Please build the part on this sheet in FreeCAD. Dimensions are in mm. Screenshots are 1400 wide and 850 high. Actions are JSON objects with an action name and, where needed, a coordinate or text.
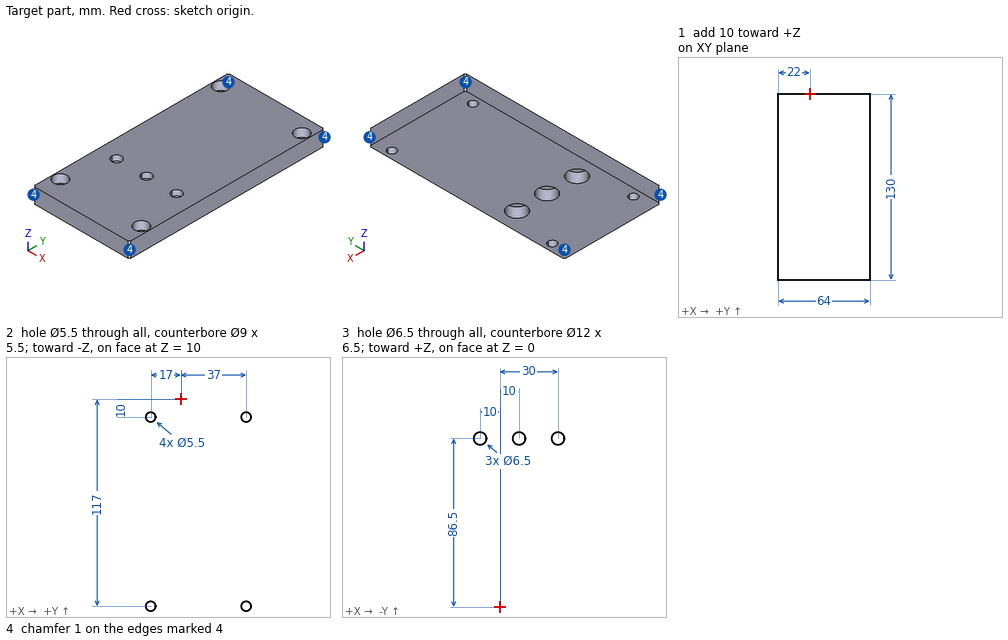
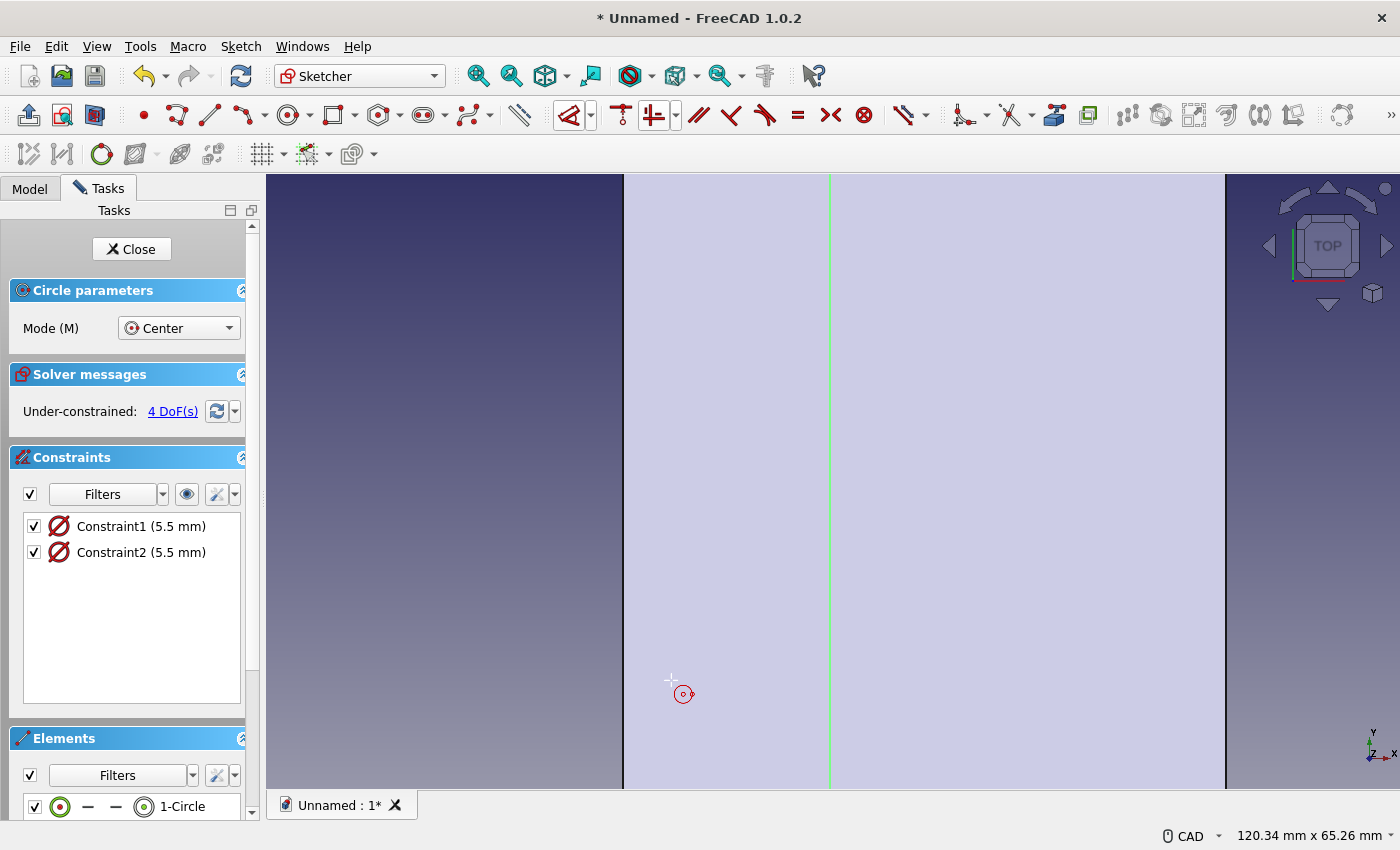
{"action": "left_click", "coordinate": [670, 678]}
{"action": "mouse_move", "coordinate": [688, 660]}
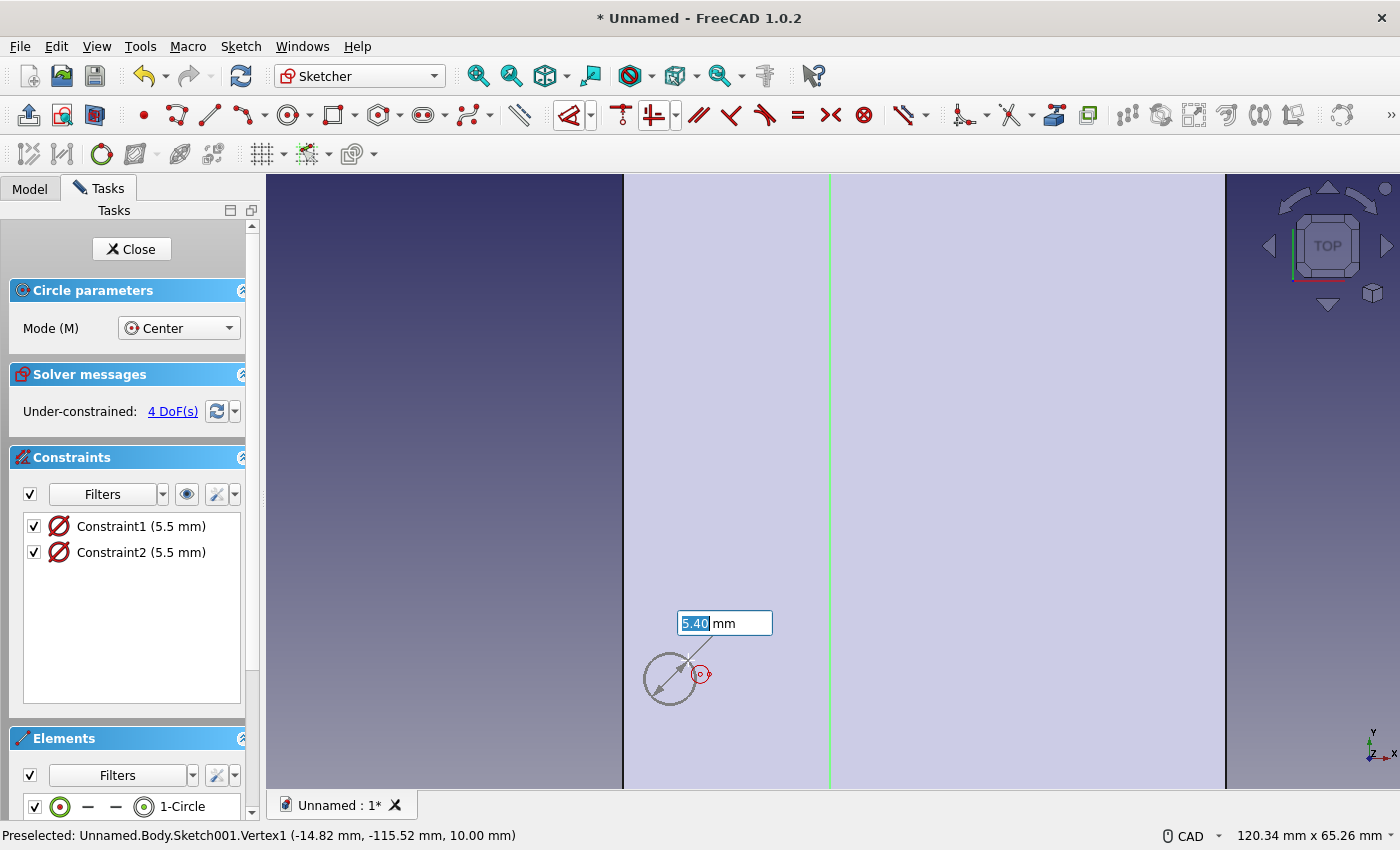
{"action": "type", "text": "5.5"}
{"action": "key", "text": "Return"}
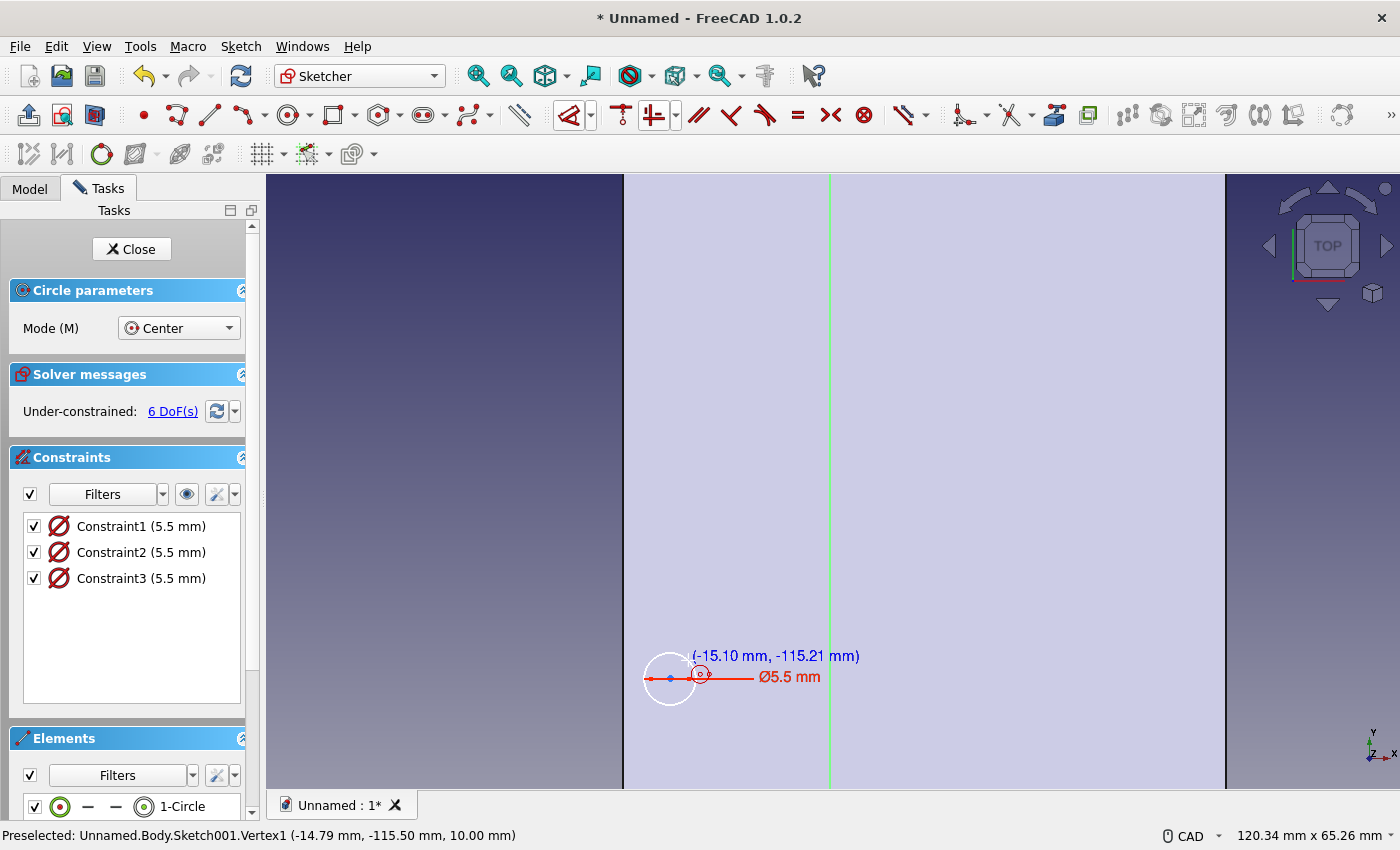
{"action": "left_click", "coordinate": [1179, 678]}
{"action": "mouse_move", "coordinate": [1197, 660]}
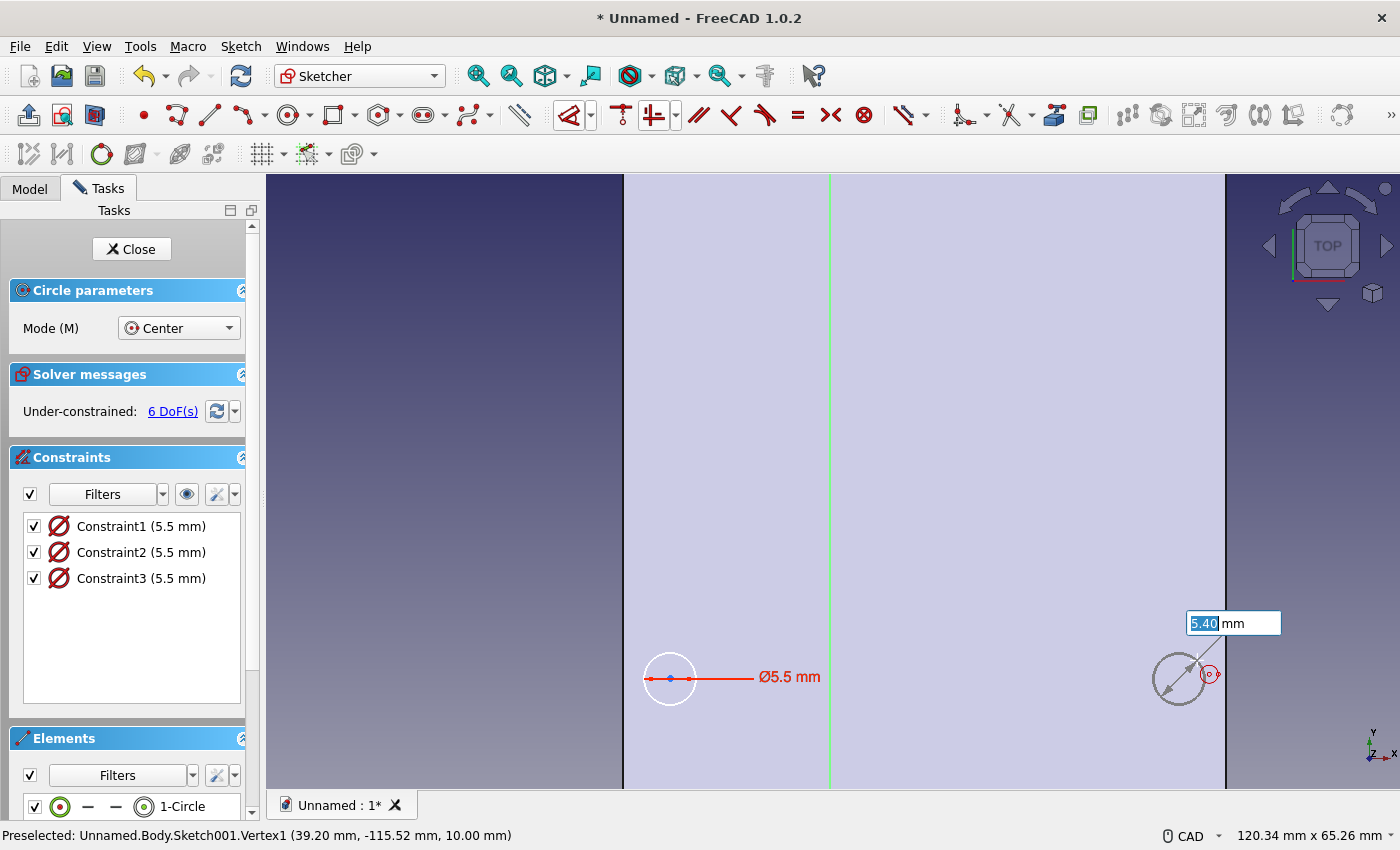
{"action": "type", "text": "5.5"}
{"action": "key", "text": "Return"}
{"action": "key", "text": "Escape"}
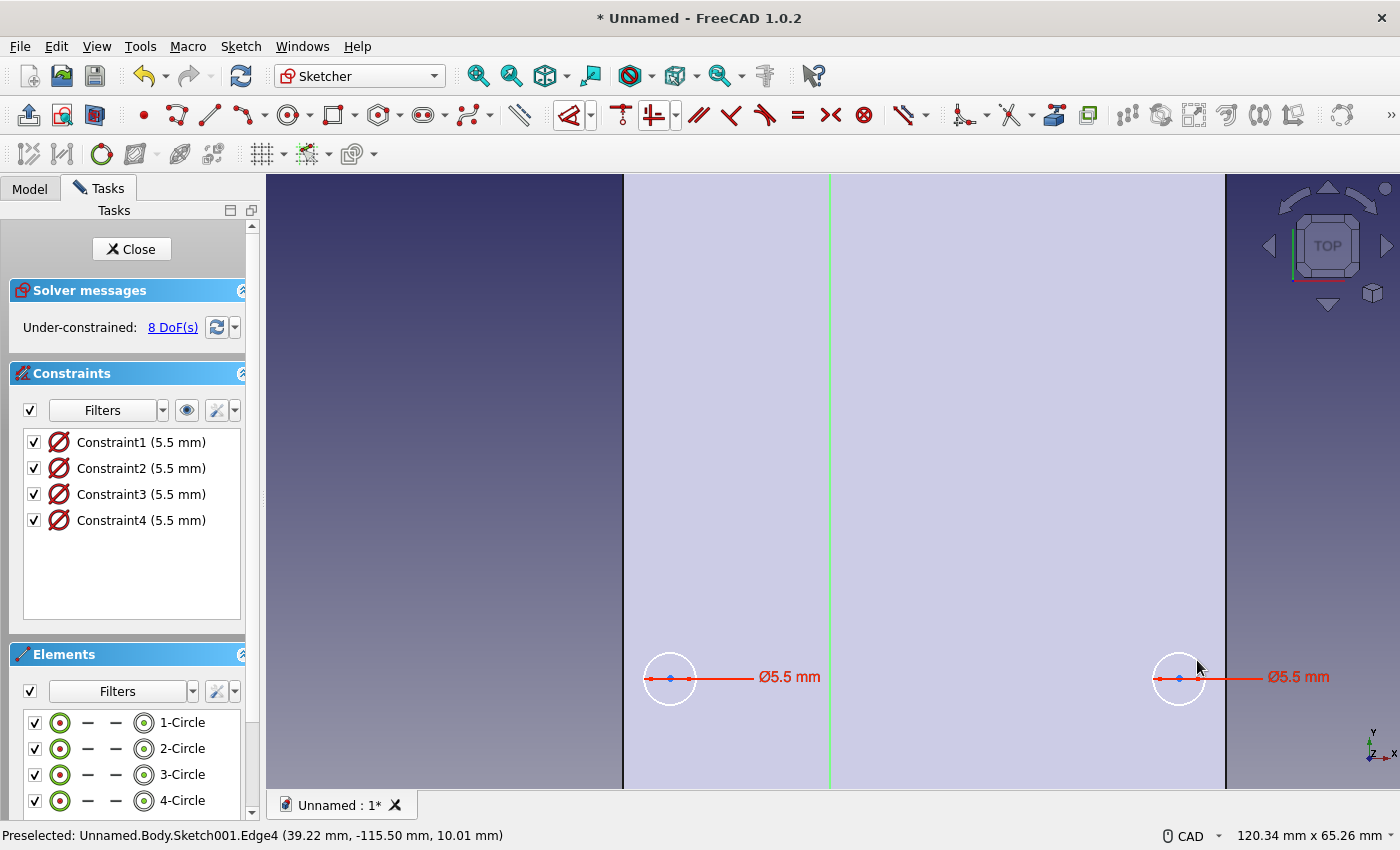
{"action": "scroll", "coordinate": [671, 680], "scroll_direction": "down", "scroll_amount": 5}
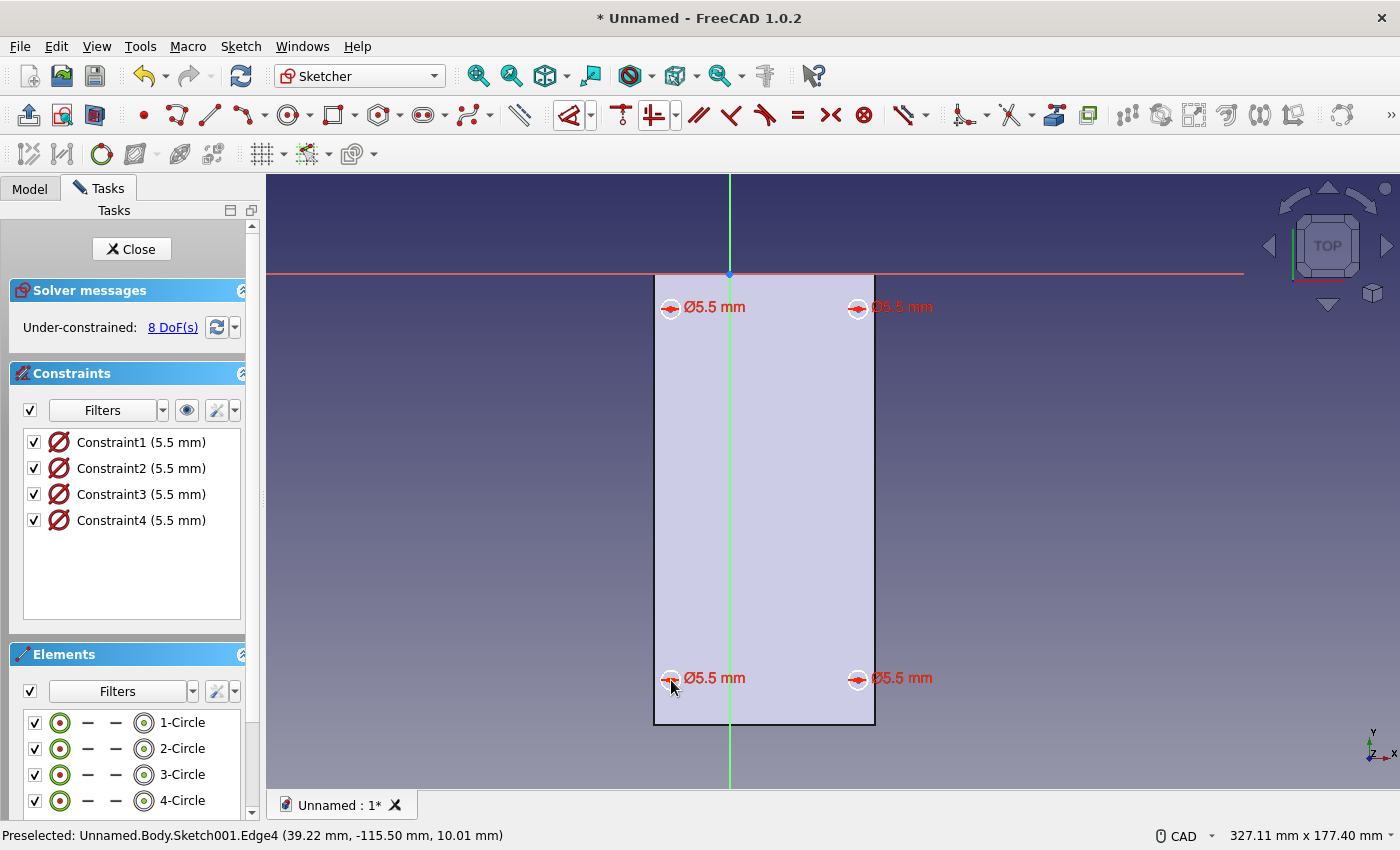
{"action": "left_click", "coordinate": [671, 309]}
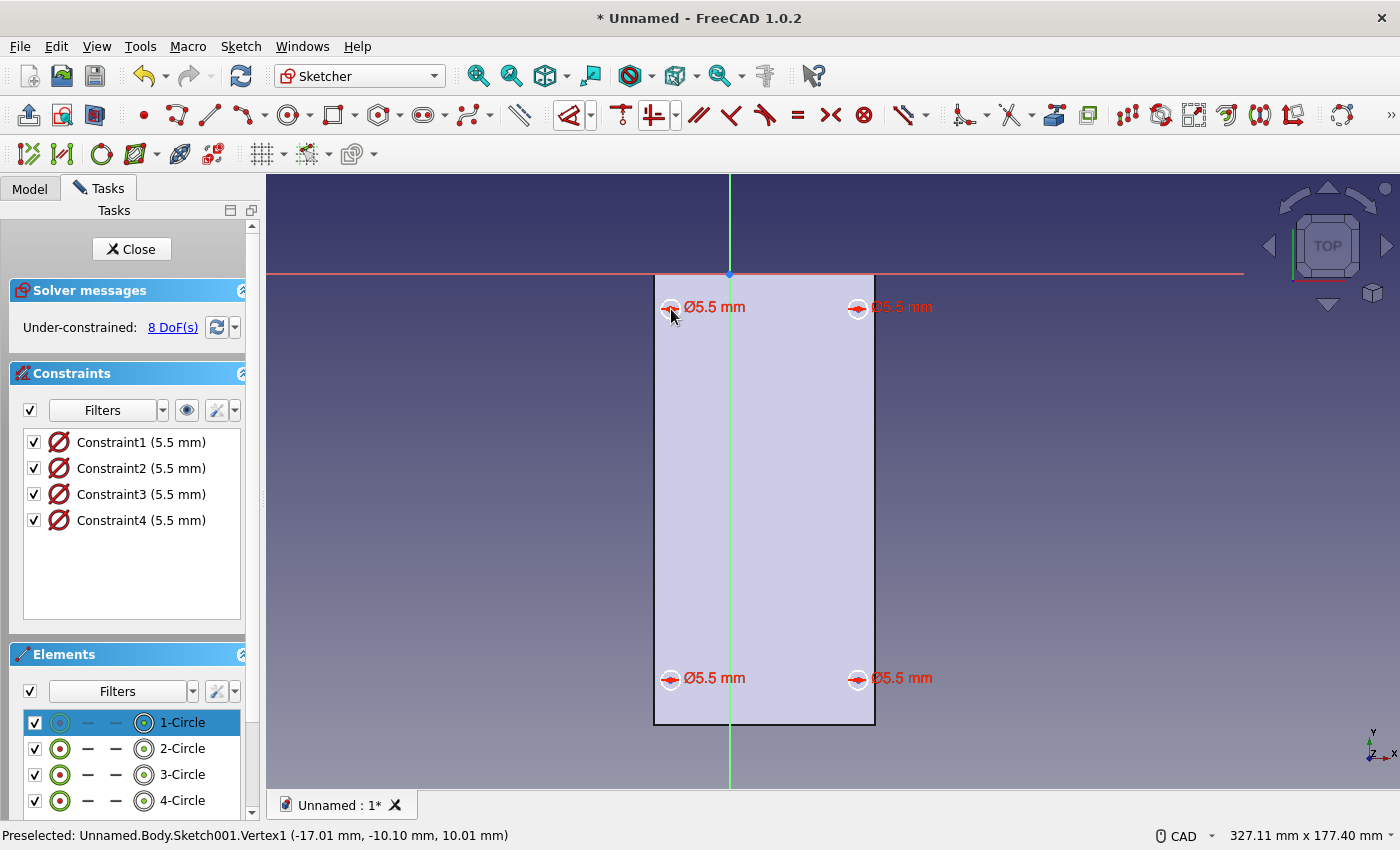
{"action": "left_click", "coordinate": [858, 309]}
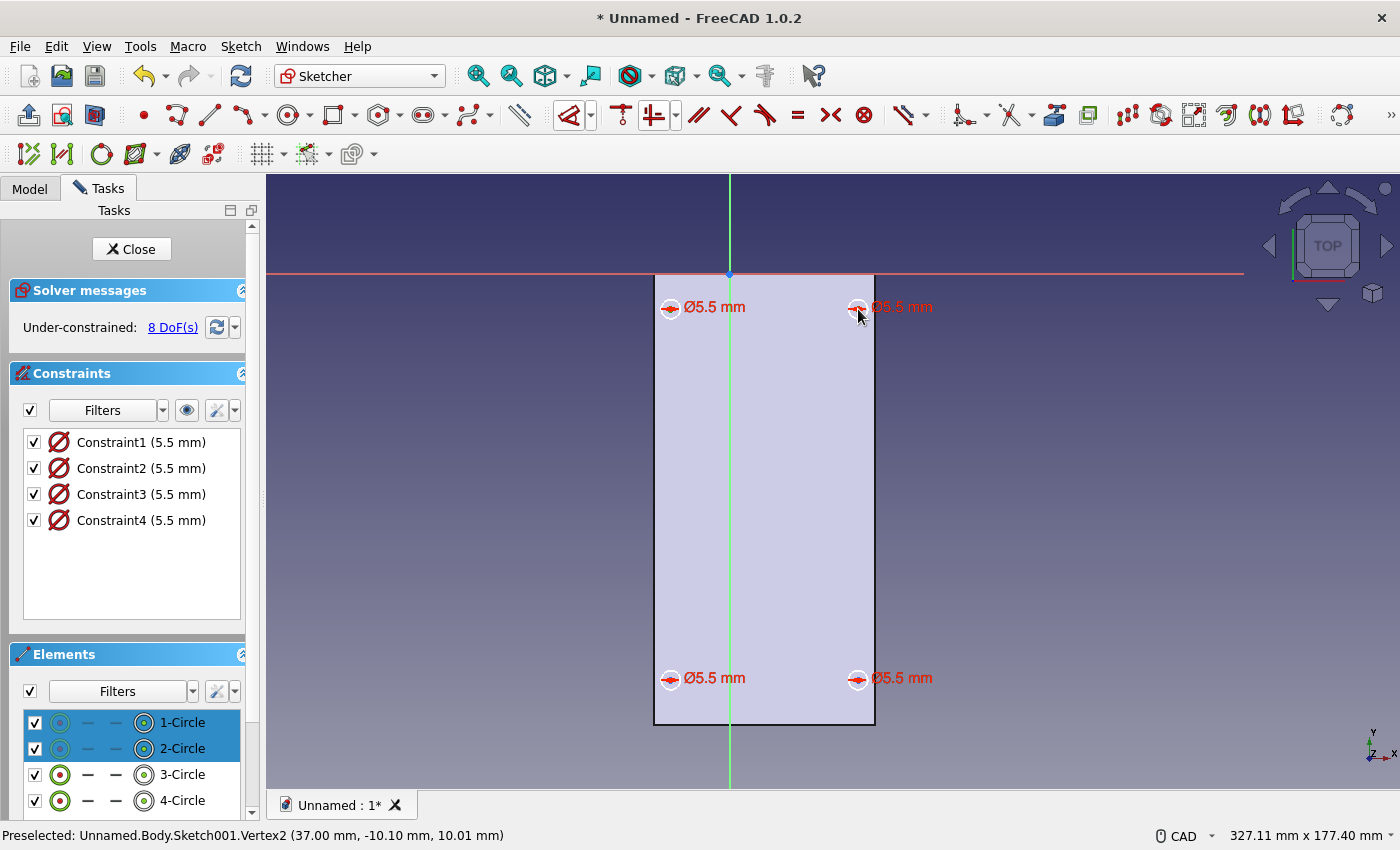
{"action": "key", "text": "h"}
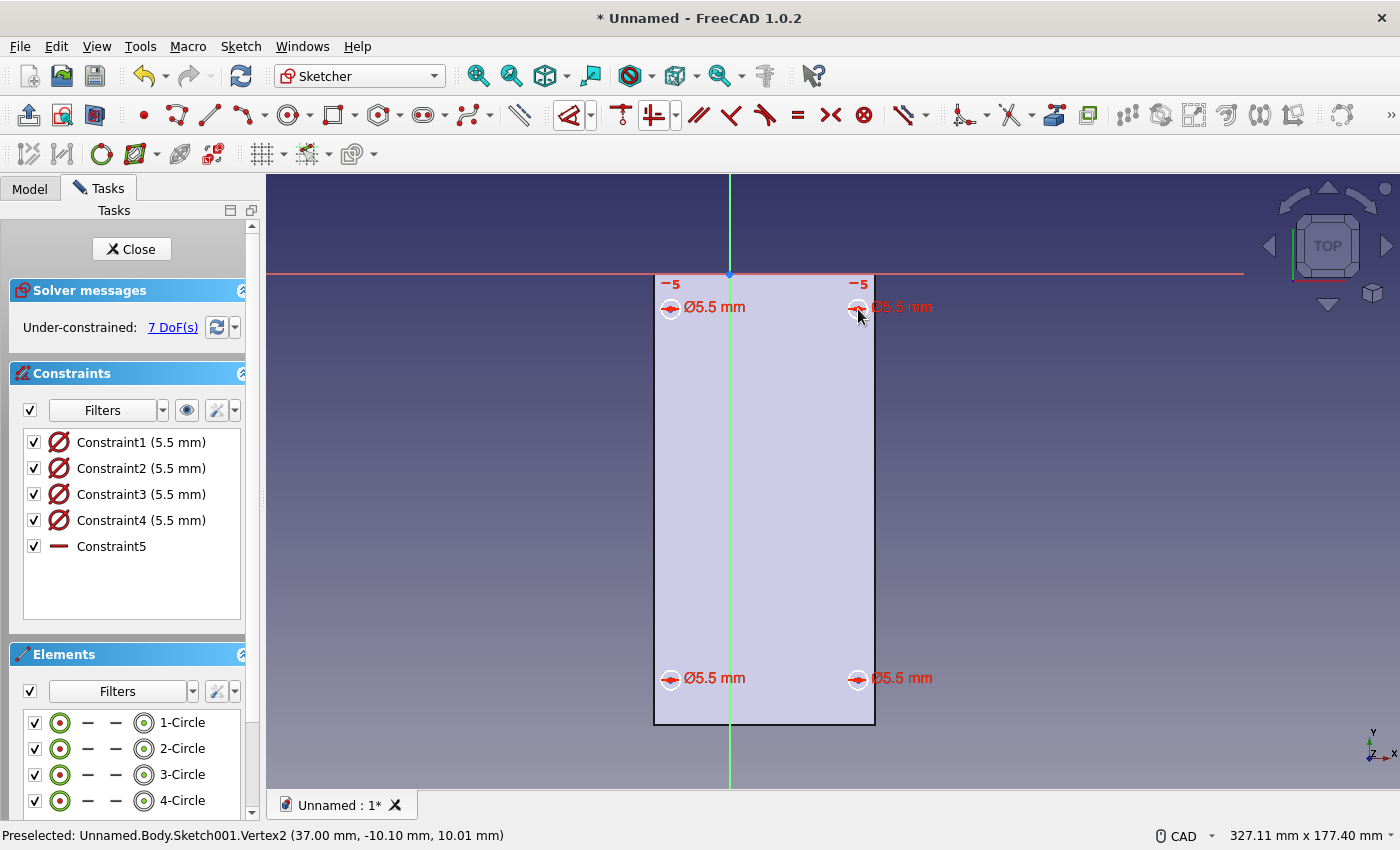
{"action": "left_click", "coordinate": [671, 309]}